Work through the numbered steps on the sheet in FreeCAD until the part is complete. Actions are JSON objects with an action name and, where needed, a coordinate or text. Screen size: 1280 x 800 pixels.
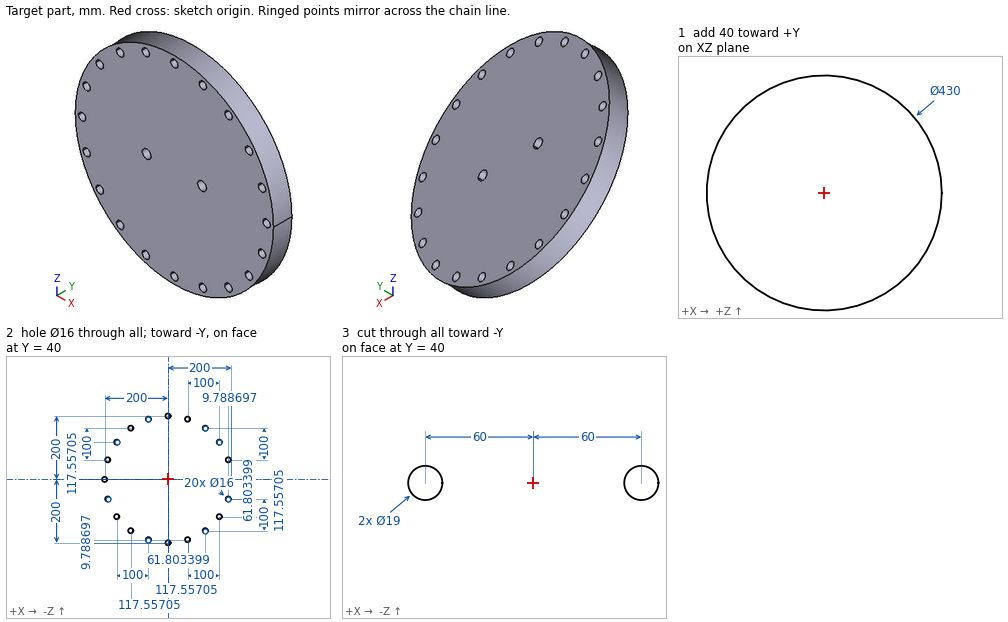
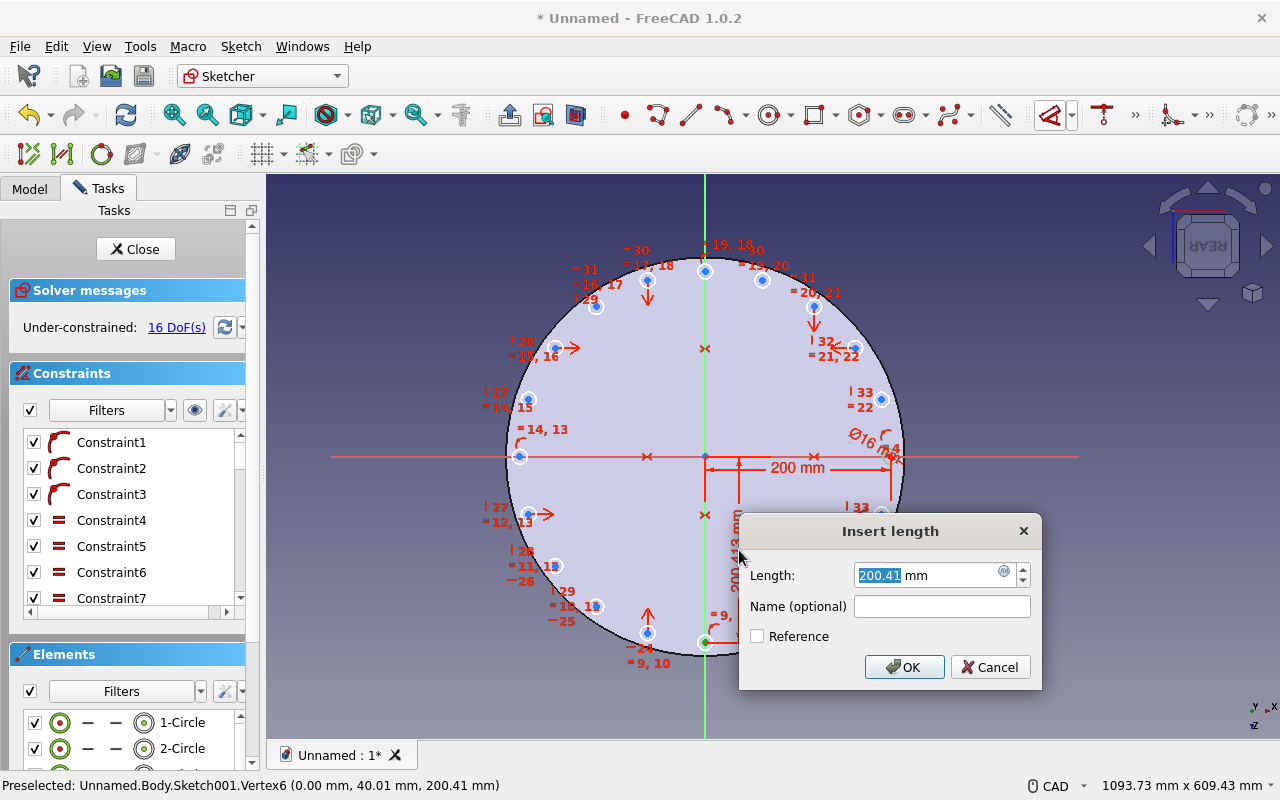
{"action": "type", "text": "200"}
{"action": "key", "text": "Return"}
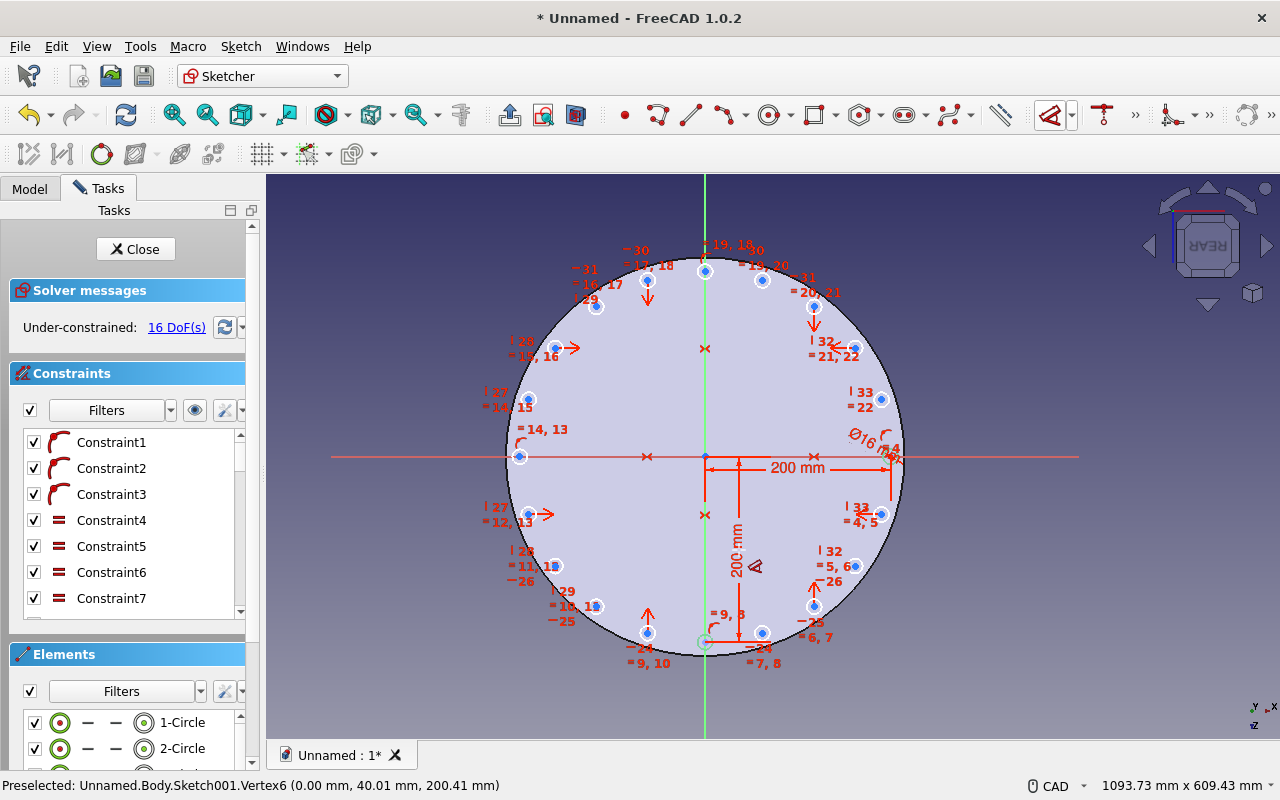
{"action": "left_click", "coordinate": [520, 457]}
{"action": "left_click", "coordinate": [613, 491]}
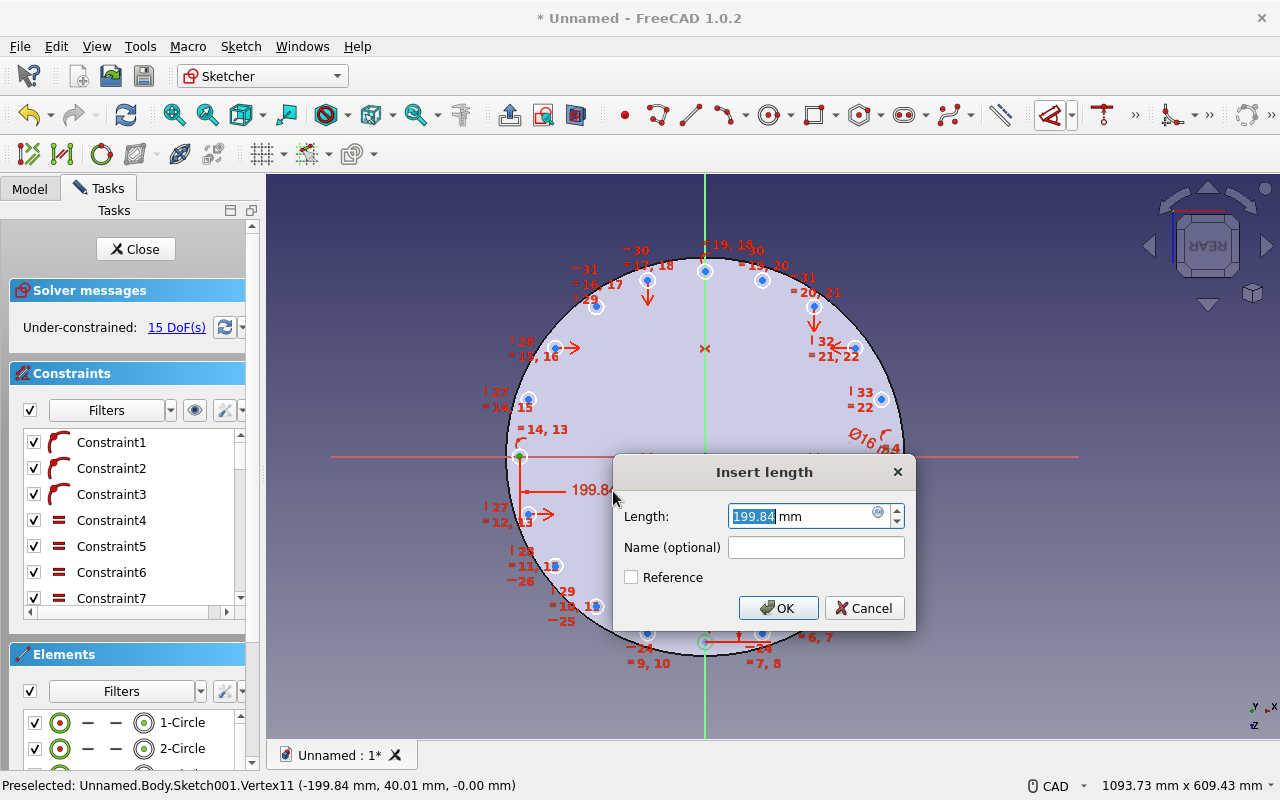
{"action": "type", "text": "200"}
{"action": "key", "text": "Return"}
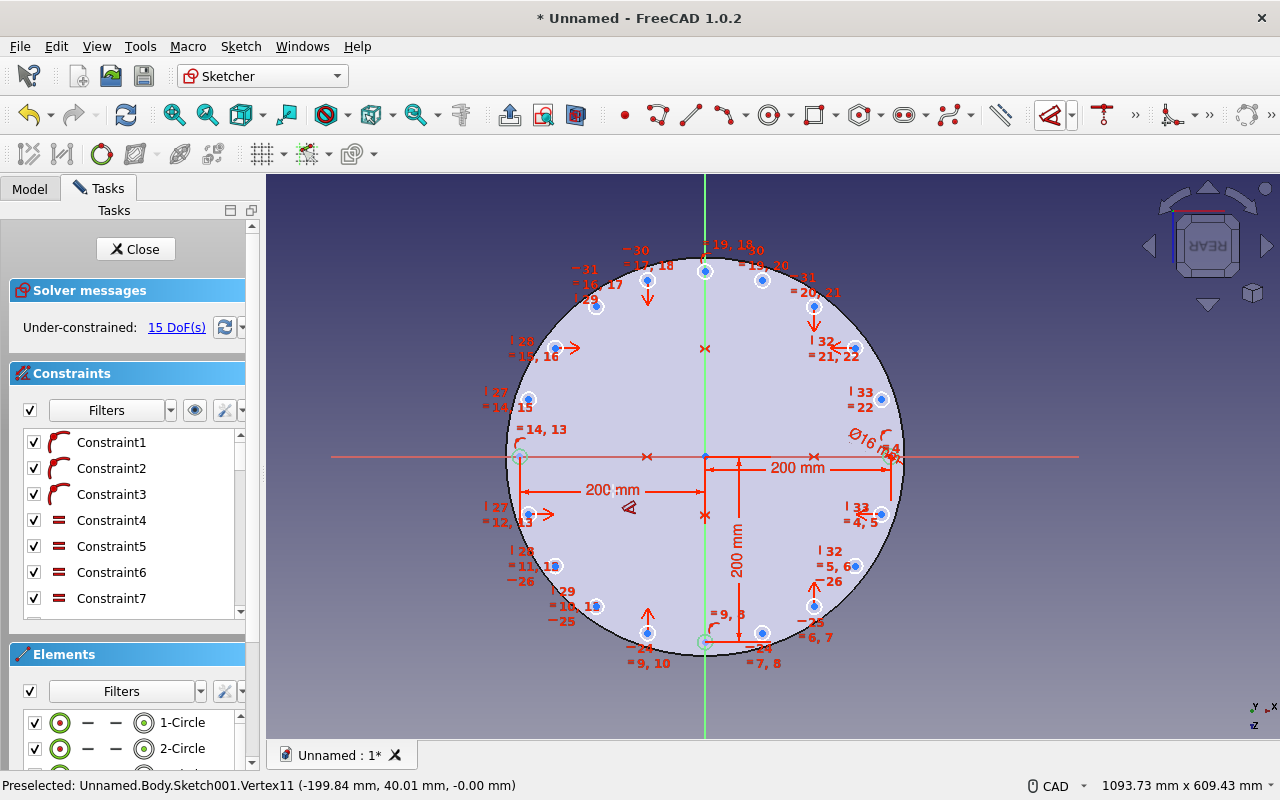
{"action": "left_click", "coordinate": [705, 272]}
{"action": "left_click", "coordinate": [739, 364]}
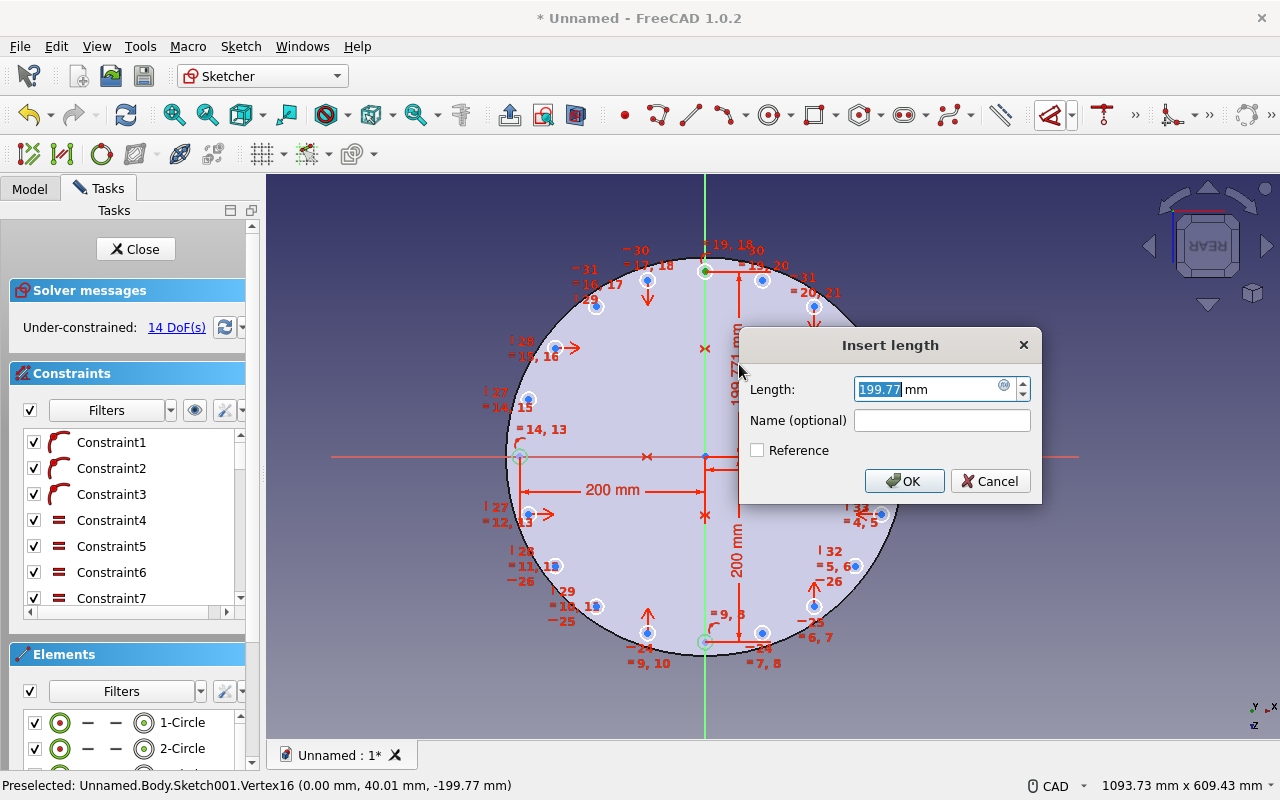
{"action": "type", "text": "200"}
{"action": "key", "text": "Return"}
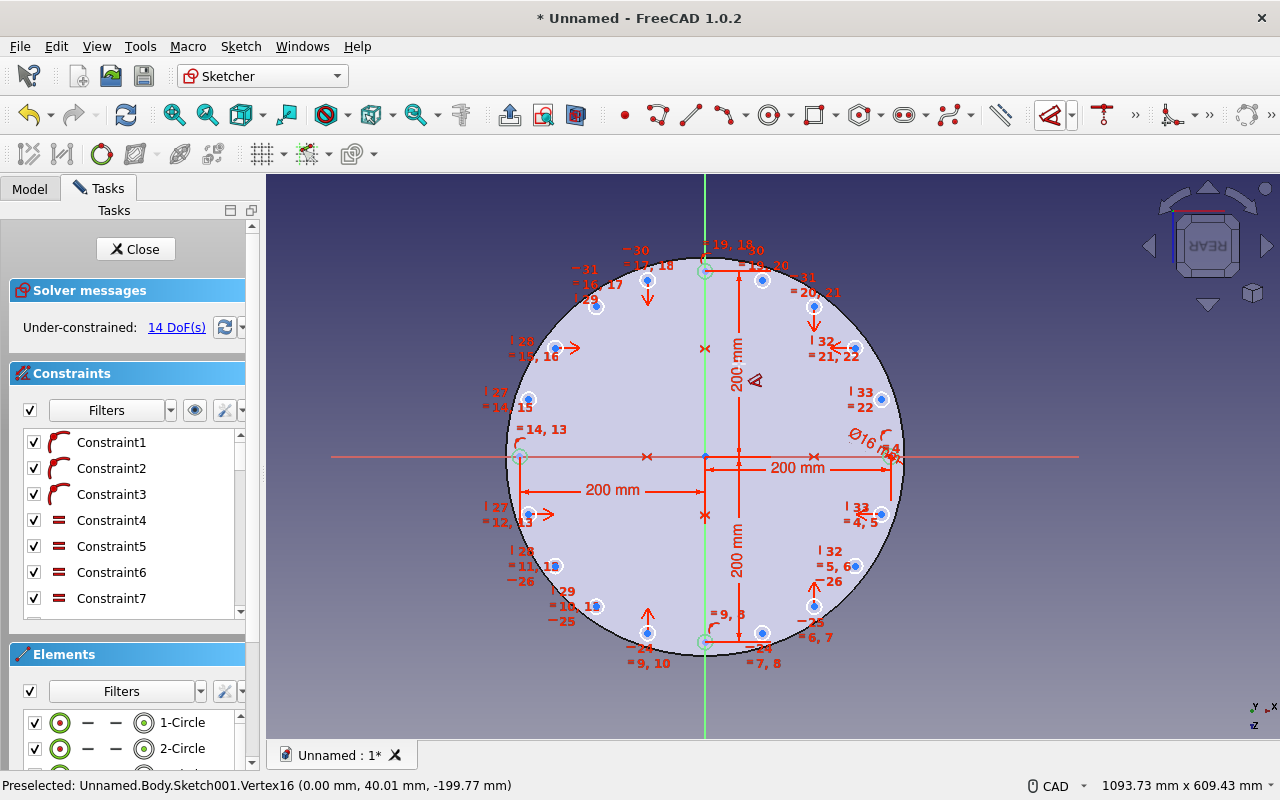
{"action": "left_click", "coordinate": [882, 514]}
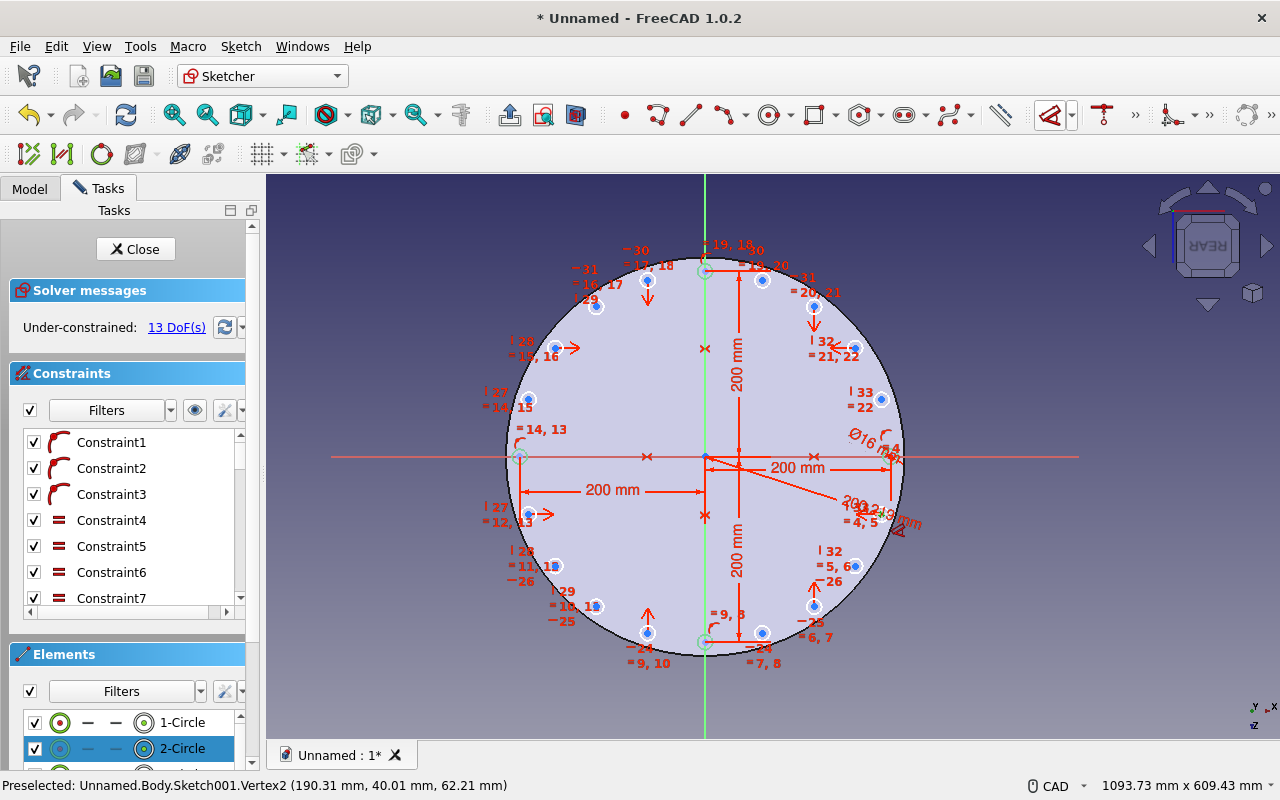
{"action": "left_click", "coordinate": [814, 607]}
{"action": "left_click", "coordinate": [916, 561]}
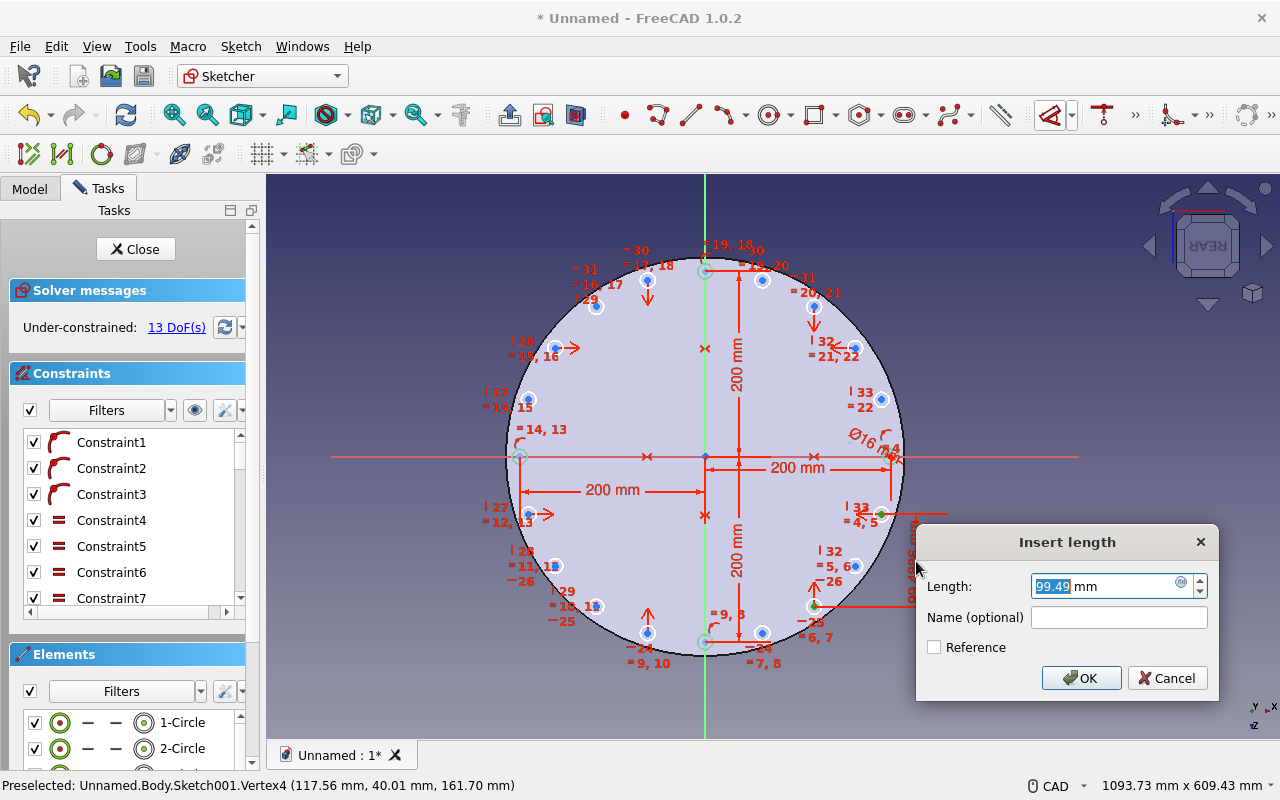
{"action": "type", "text": "100"}
{"action": "key", "text": "Return"}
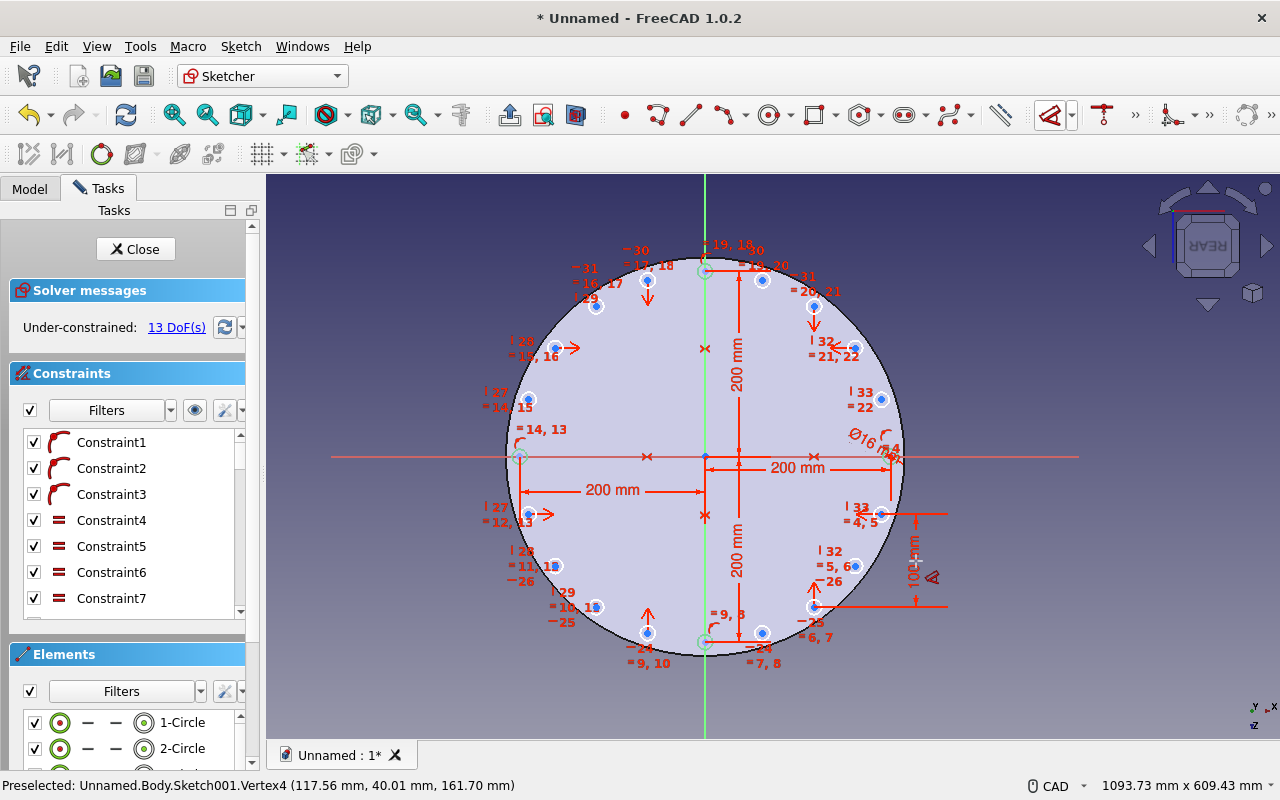
{"action": "left_click", "coordinate": [855, 566]}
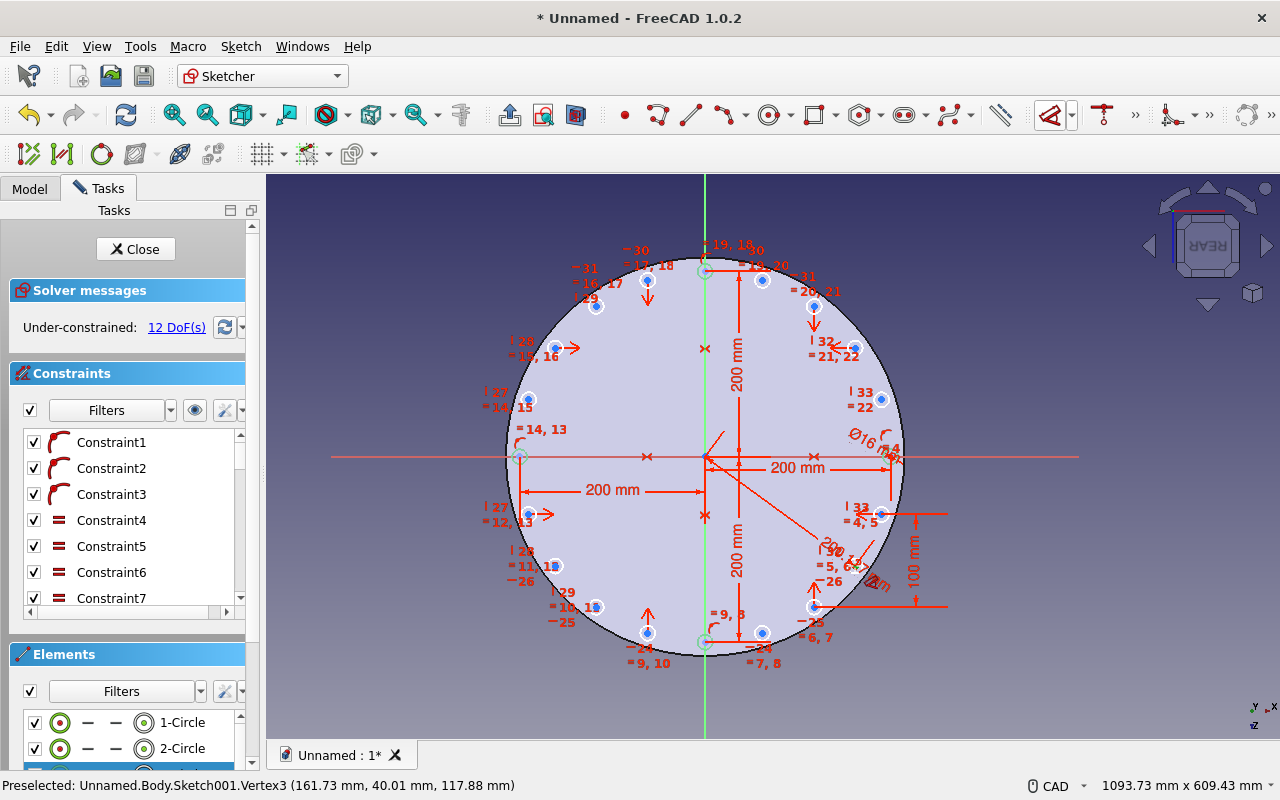
{"action": "left_click", "coordinate": [762, 633]}
{"action": "left_click", "coordinate": [809, 667]}